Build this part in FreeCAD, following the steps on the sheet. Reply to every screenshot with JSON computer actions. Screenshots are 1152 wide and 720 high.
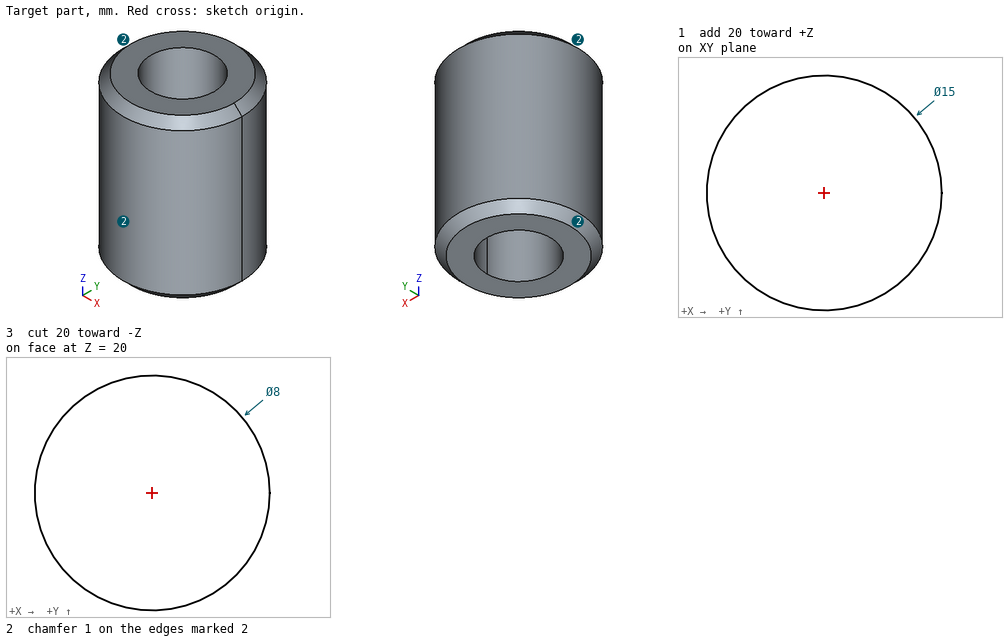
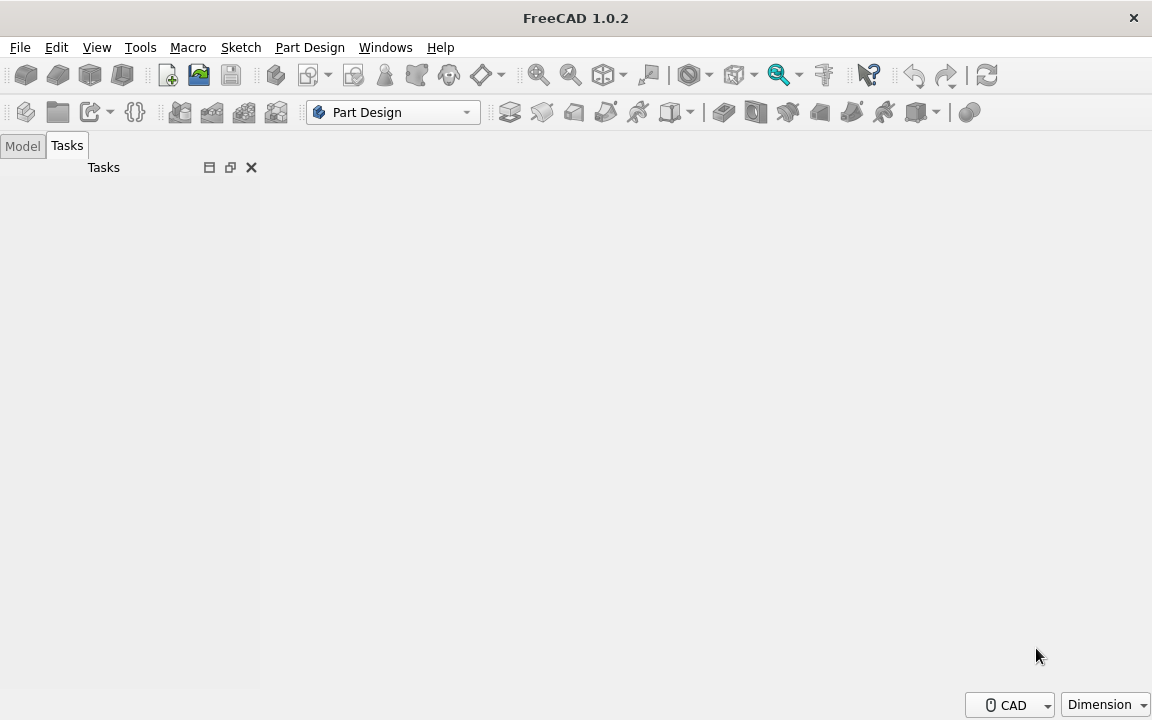
{"action": "key", "text": "ctrl+n"}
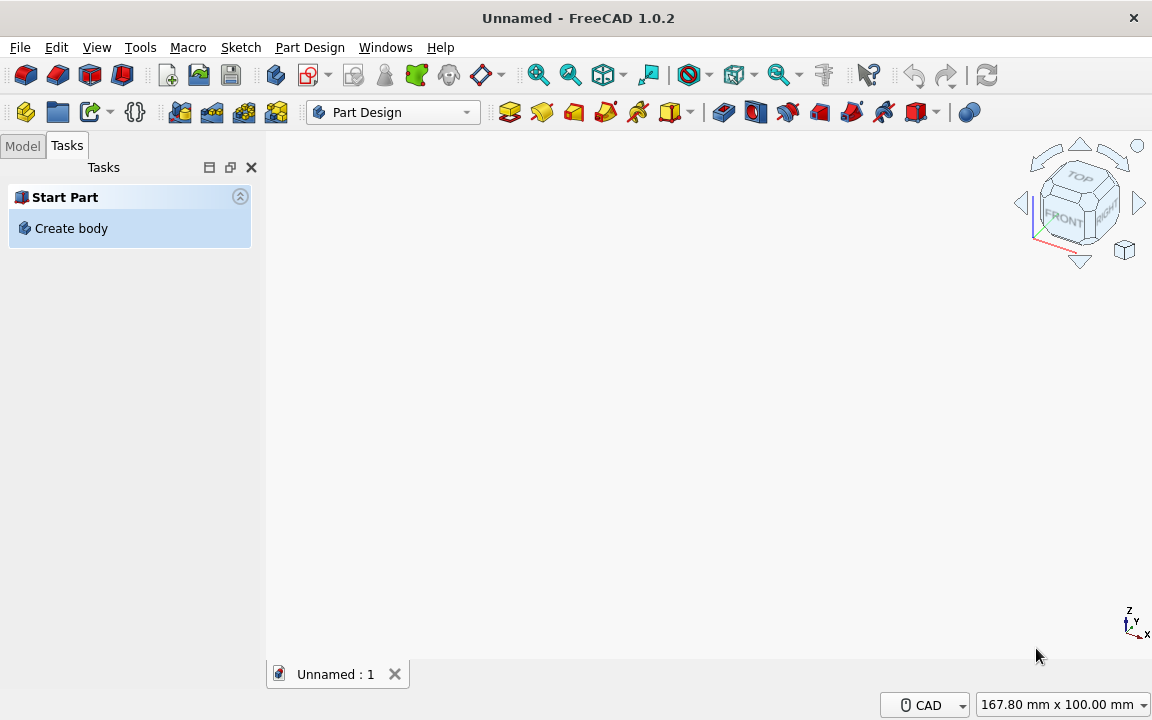
{"action": "left_click", "coordinate": [308, 76]}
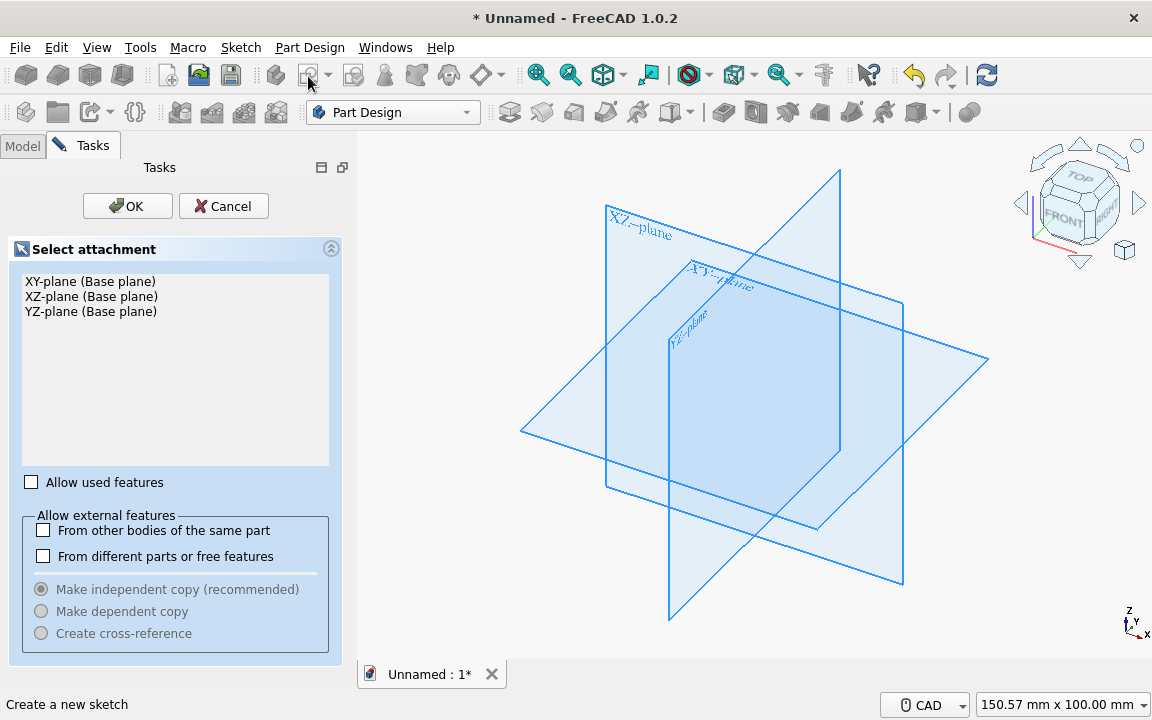
{"action": "left_click", "coordinate": [82, 282]}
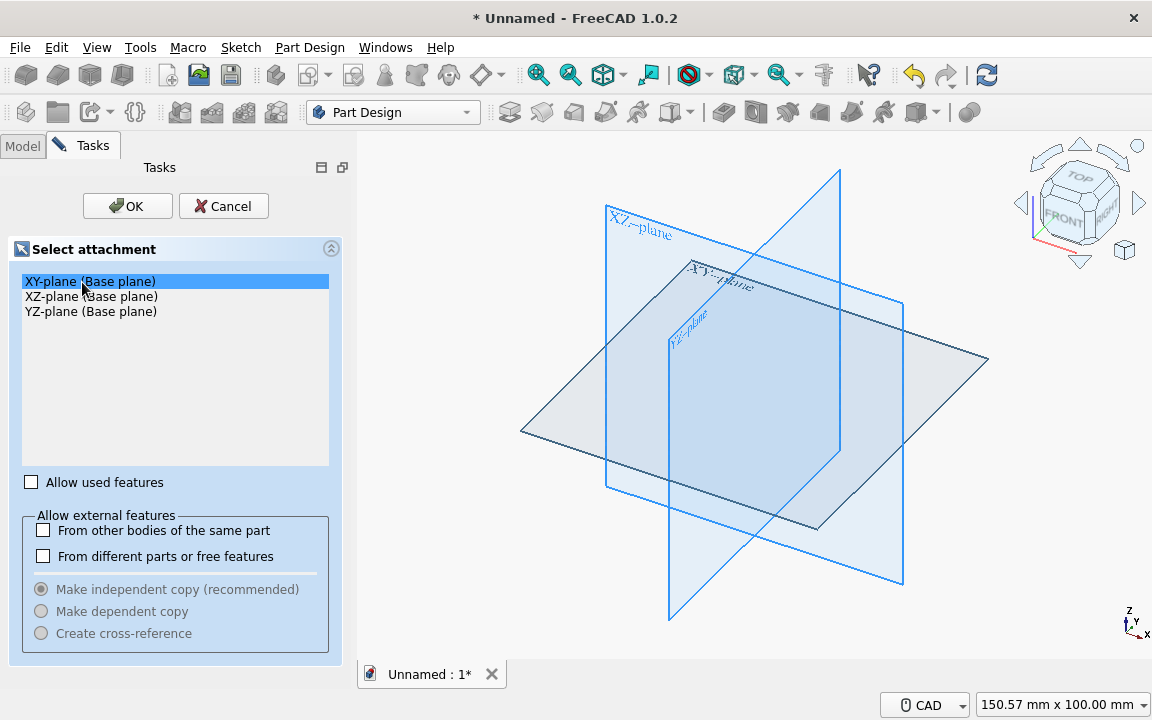
{"action": "left_click", "coordinate": [128, 206]}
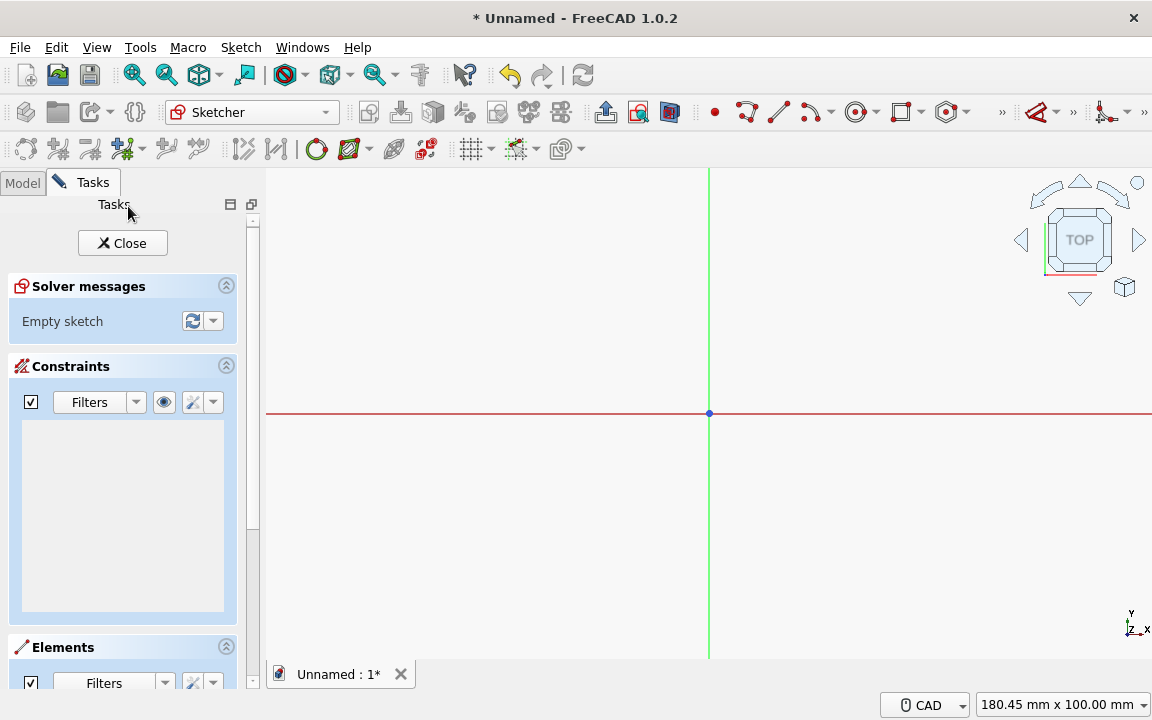
{"action": "scroll", "coordinate": [731, 414], "scroll_direction": "up", "scroll_amount": 7}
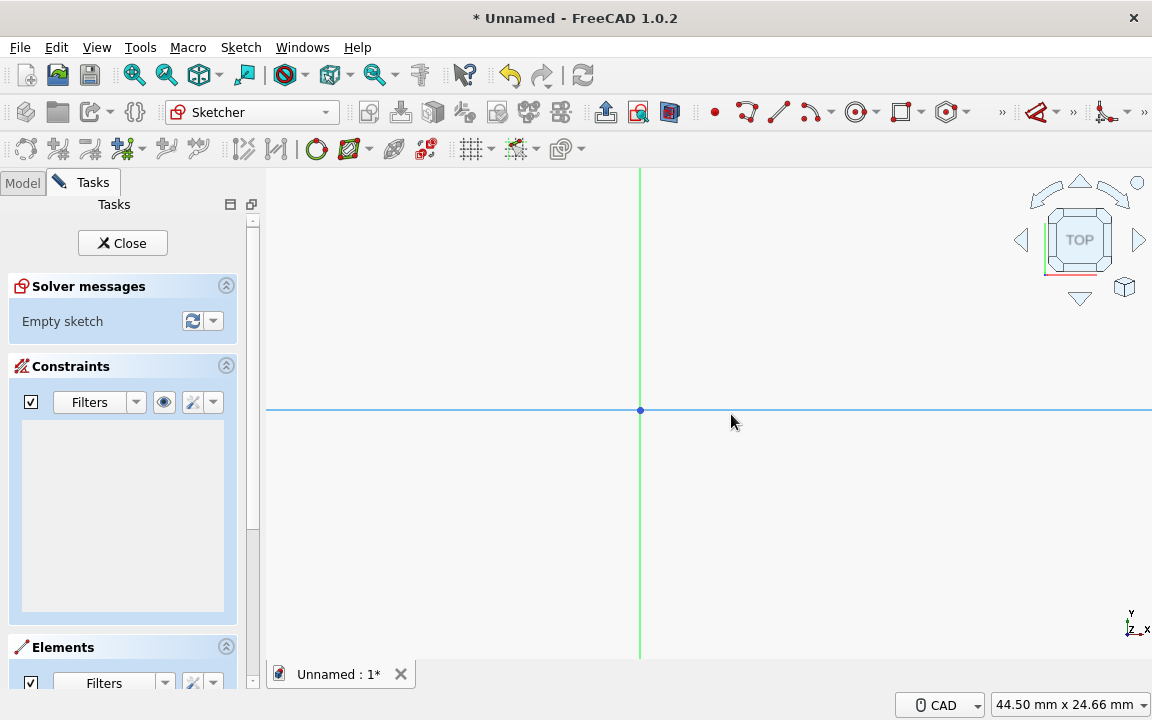
{"action": "left_click", "coordinate": [856, 112]}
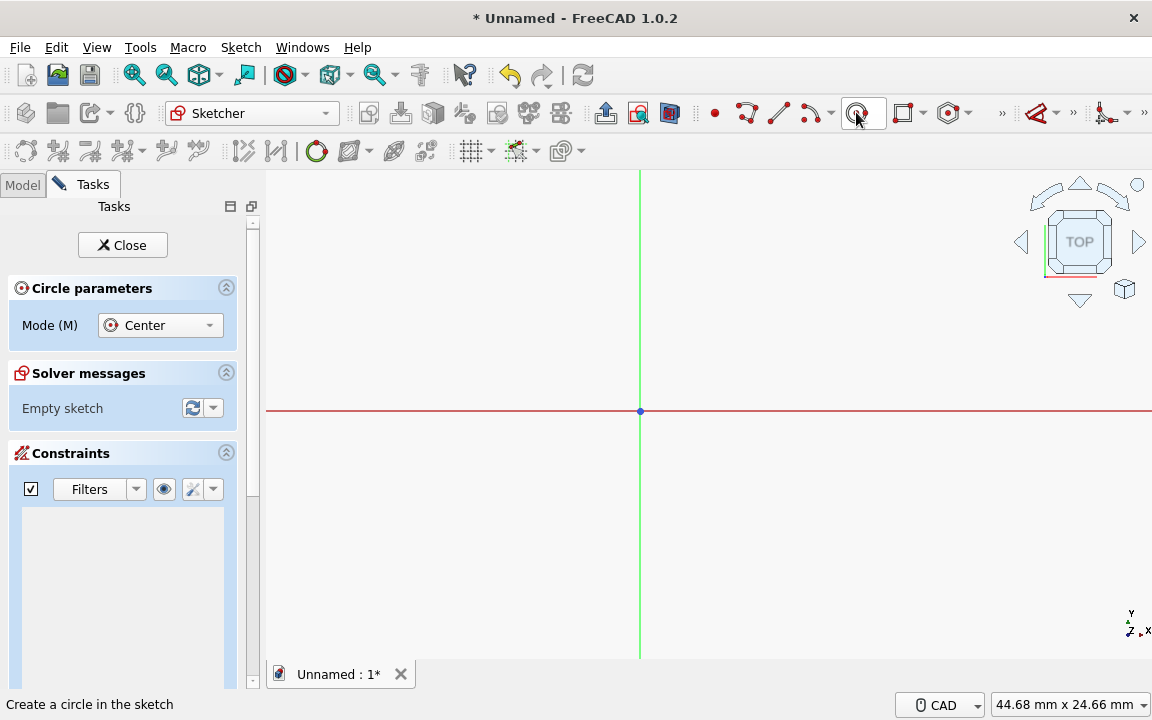
{"action": "left_click", "coordinate": [640, 411]}
{"action": "left_click", "coordinate": [746, 306]}
{"action": "key", "text": "Escape"}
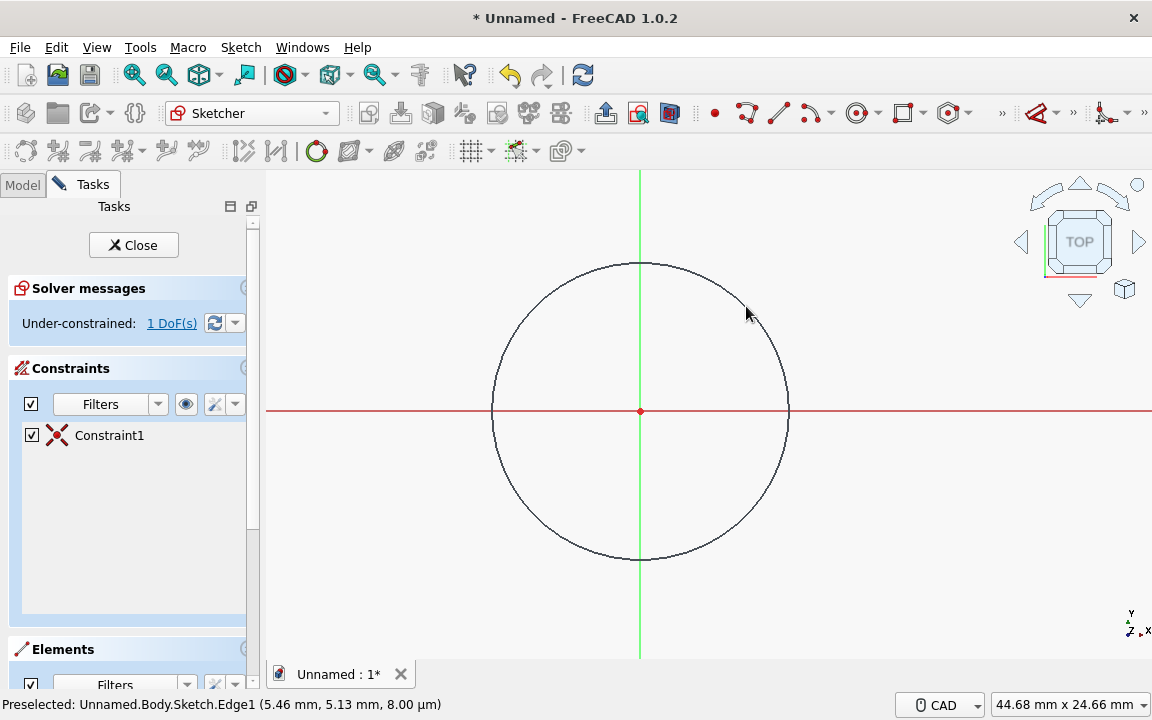
{"action": "left_click", "coordinate": [1036, 114]}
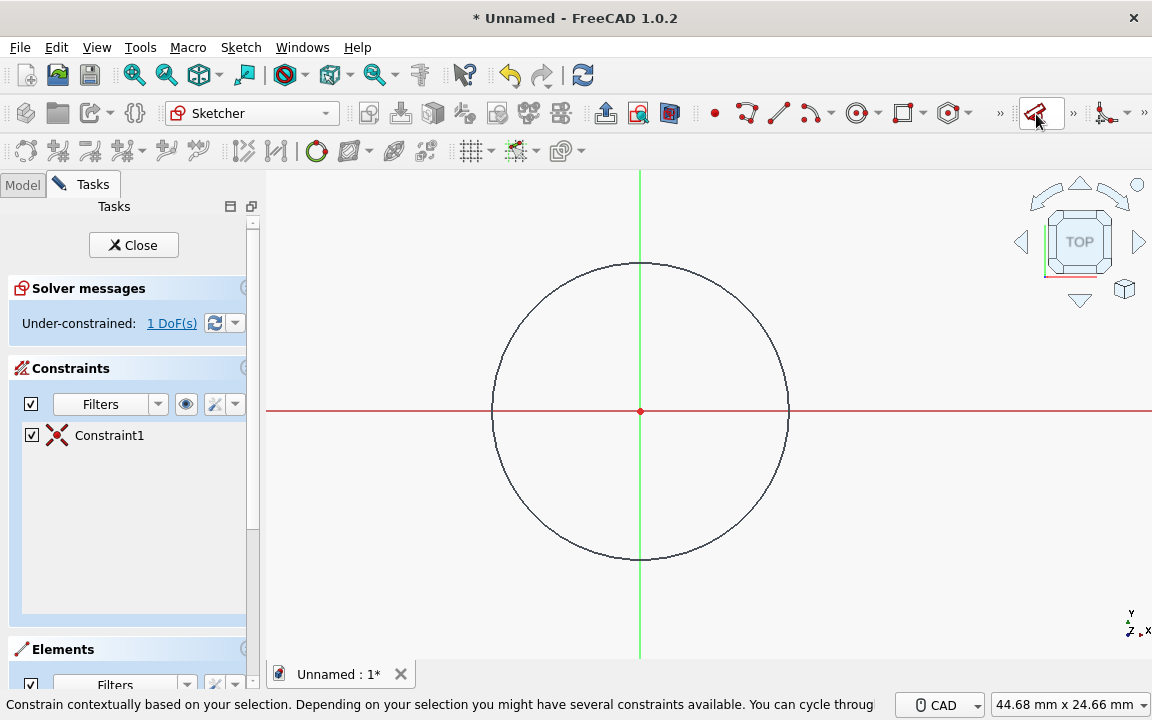
{"action": "left_click", "coordinate": [745, 306]}
{"action": "left_click", "coordinate": [768, 283]}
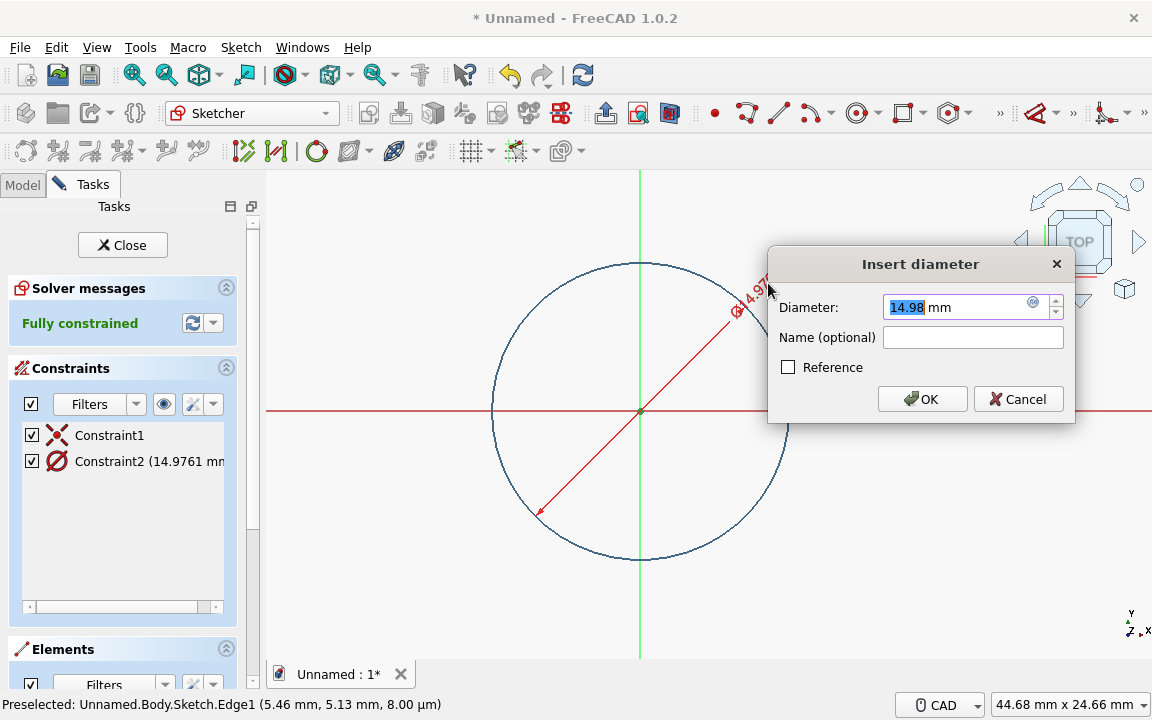
{"action": "type", "text": "15"}
{"action": "key", "text": "Return"}
{"action": "key", "text": "Escape"}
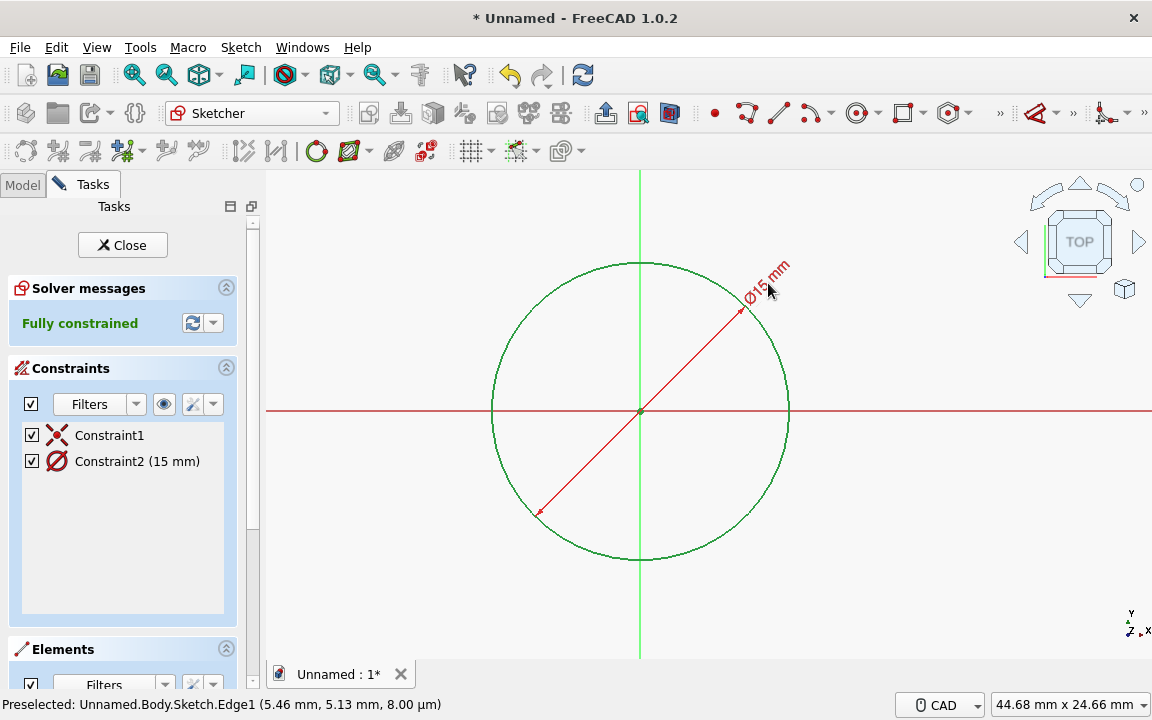
{"action": "left_click", "coordinate": [123, 245]}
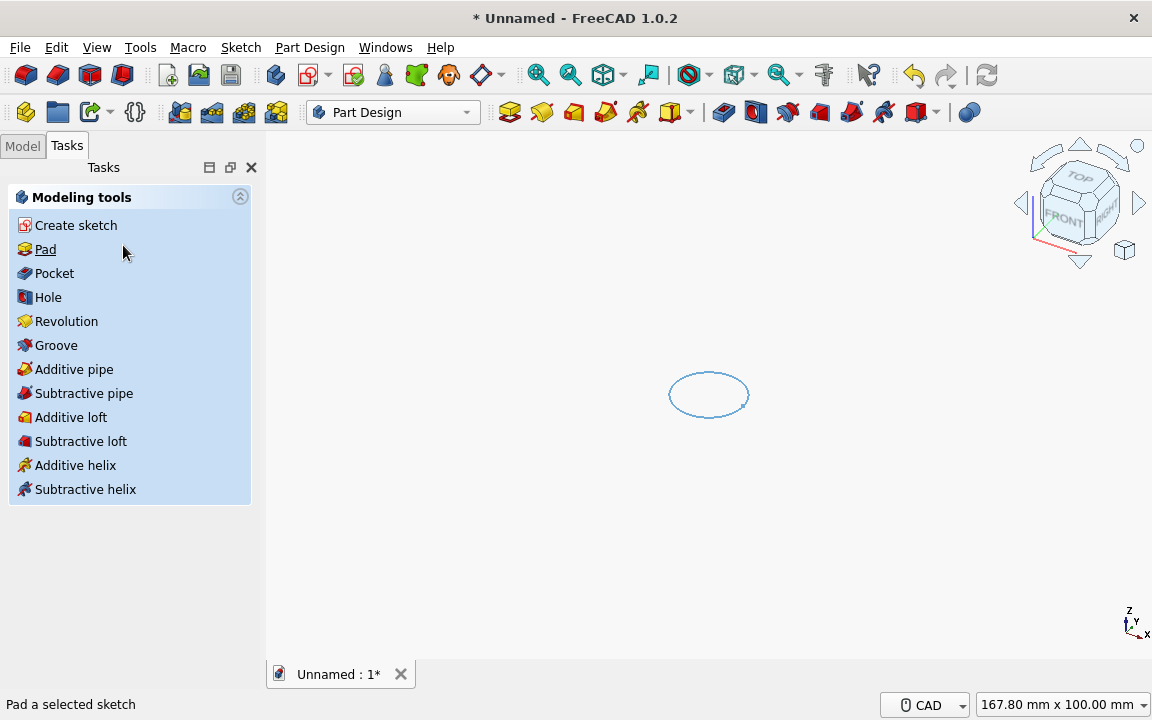
{"action": "left_click", "coordinate": [510, 112]}